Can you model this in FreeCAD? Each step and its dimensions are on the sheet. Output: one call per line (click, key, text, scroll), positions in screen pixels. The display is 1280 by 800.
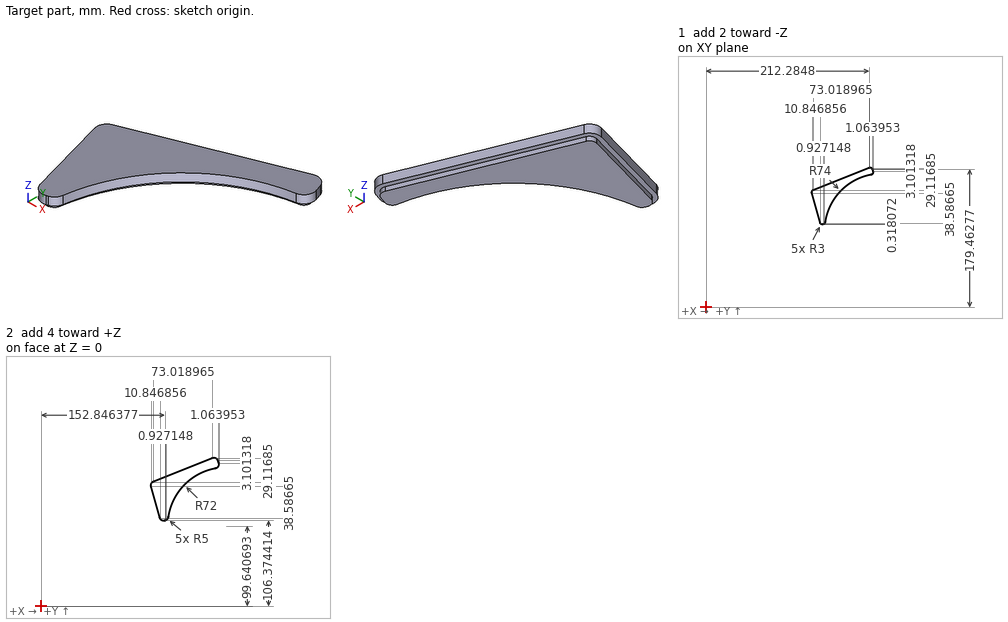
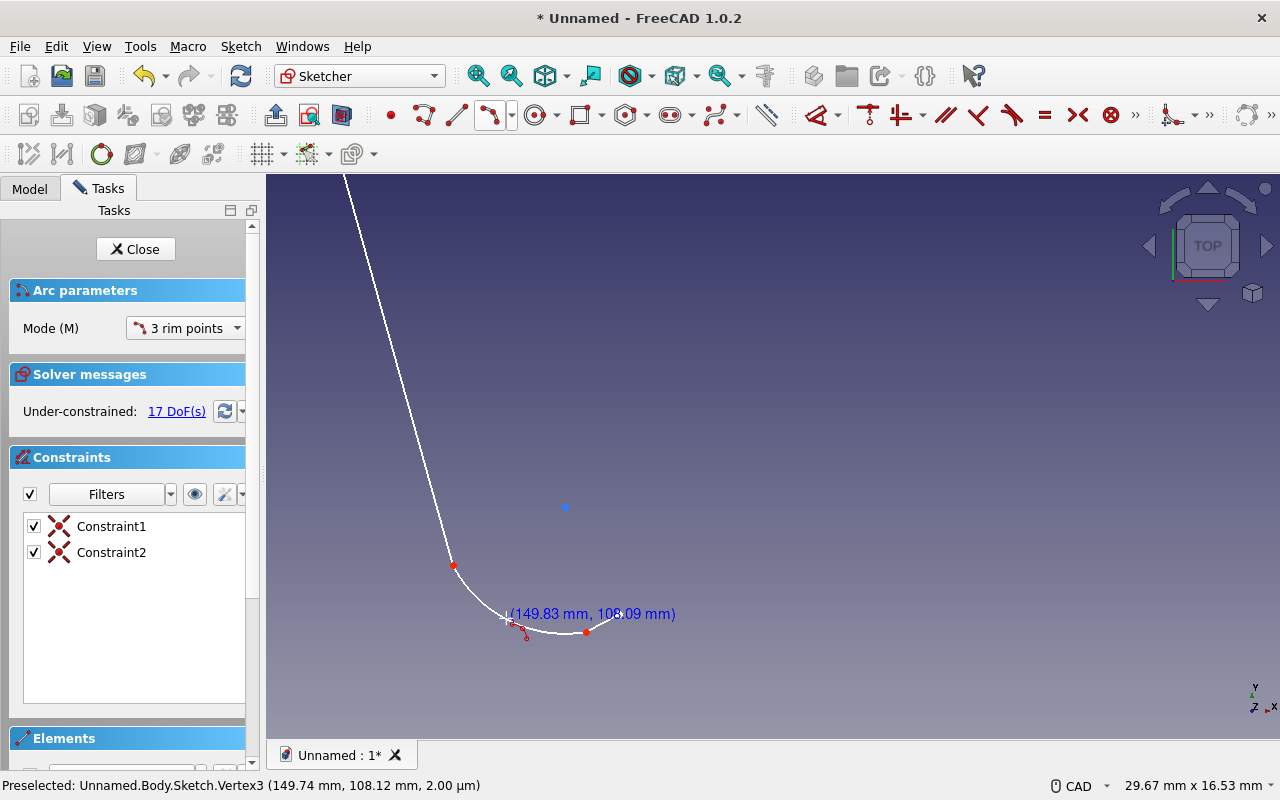
click(619, 614)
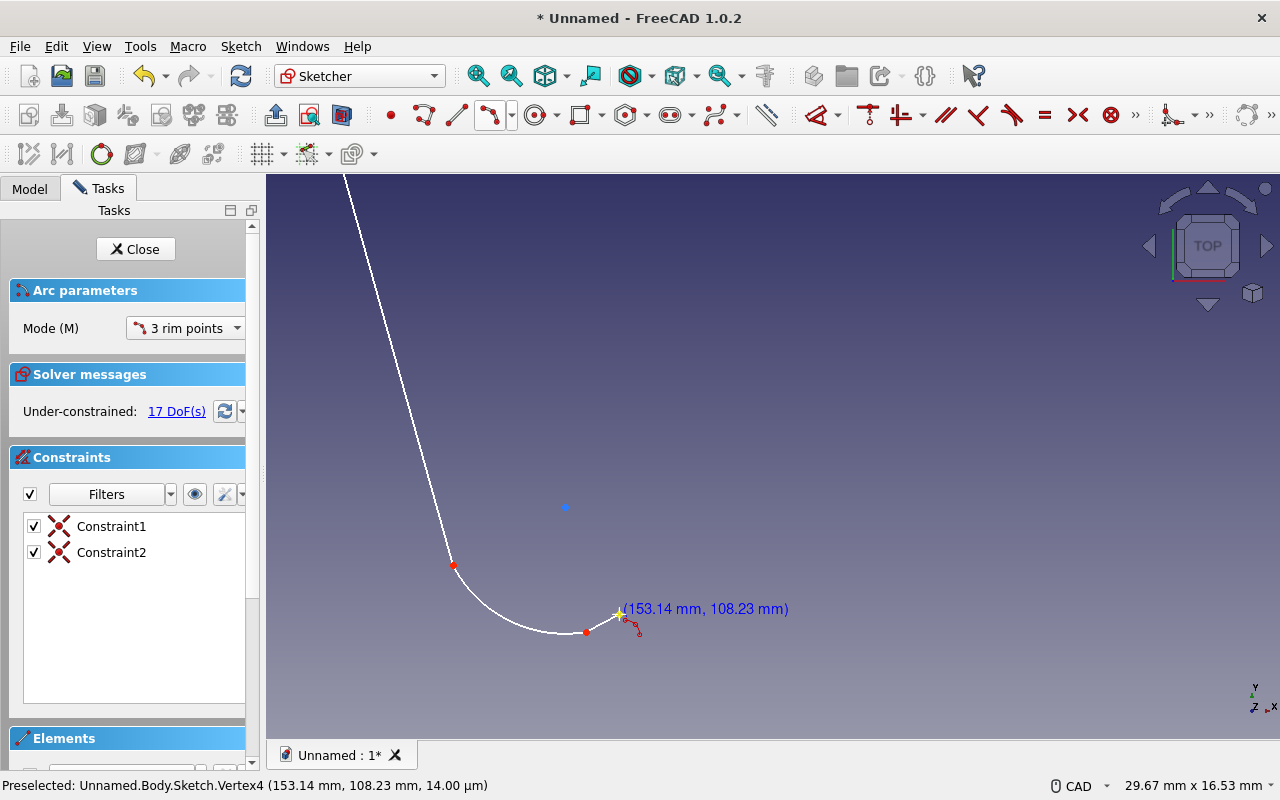
scroll(588, 626, down, 10)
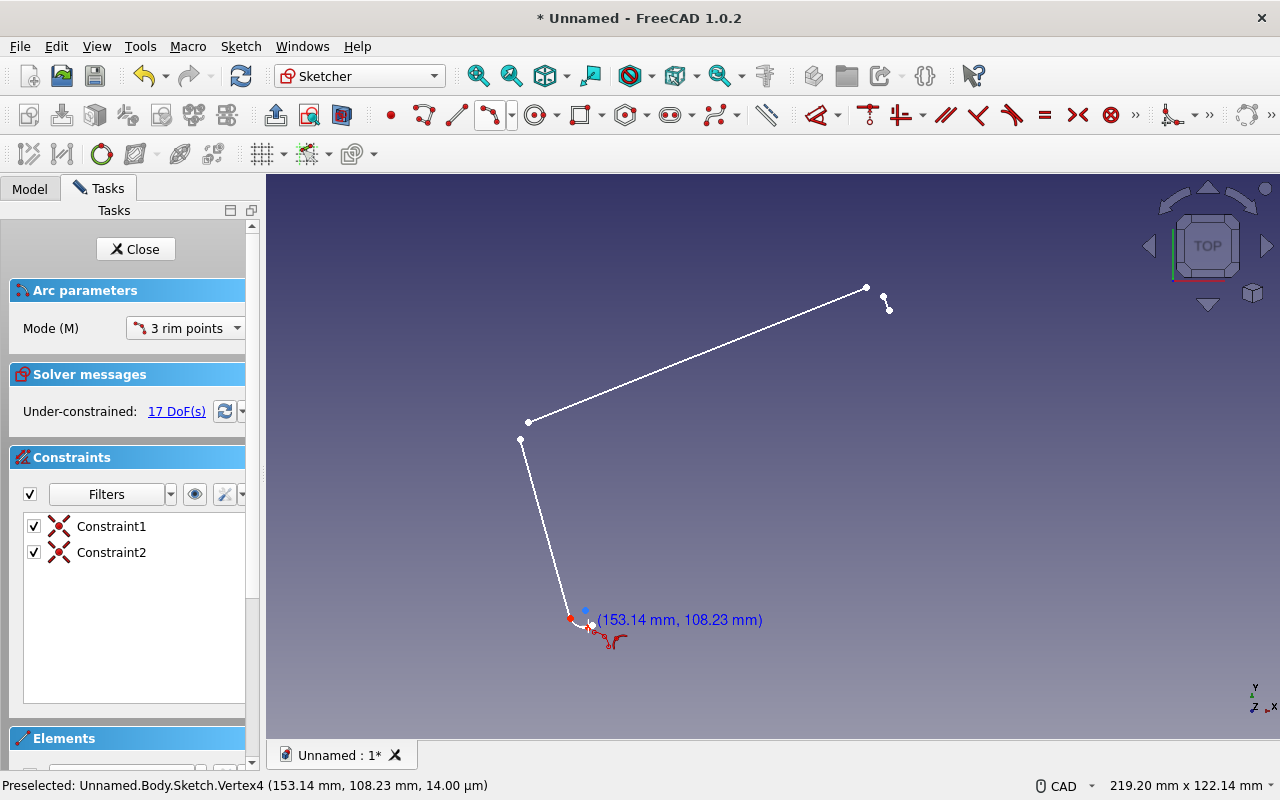
click(602, 614)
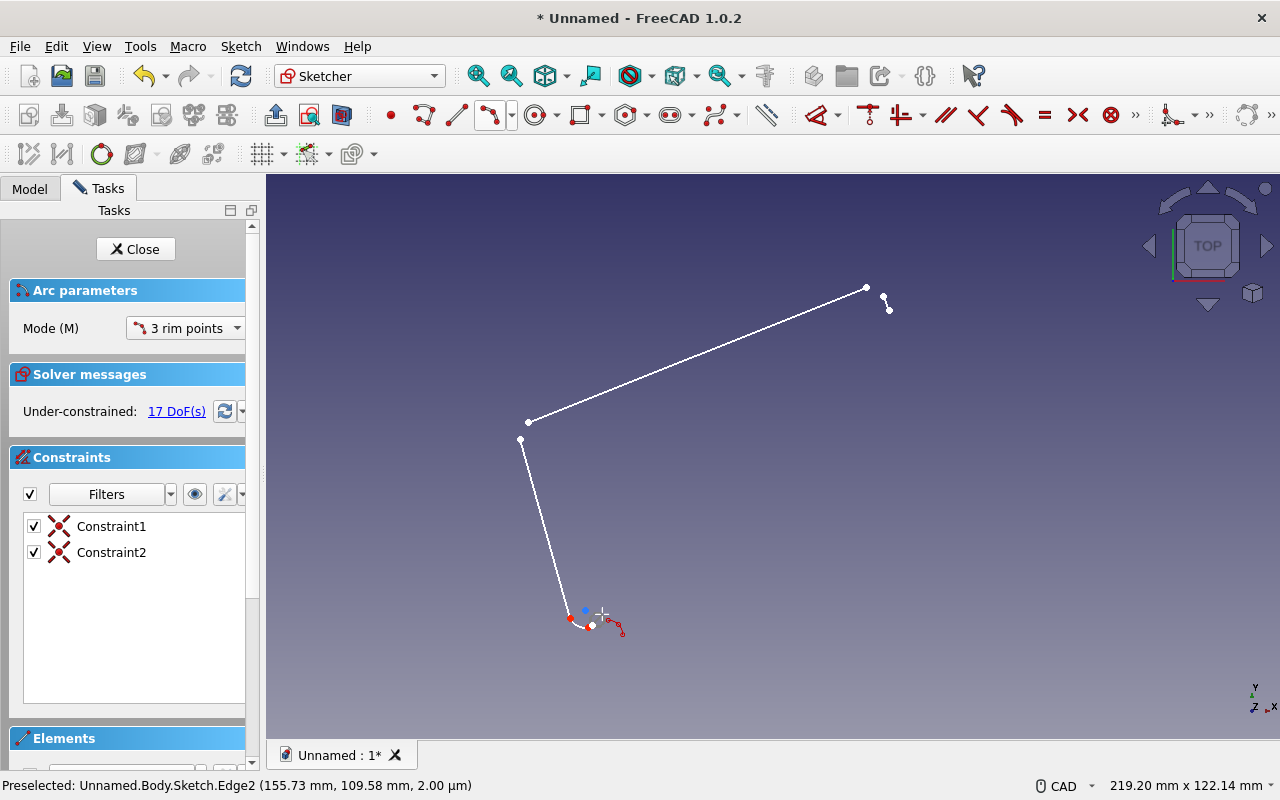
scroll(599, 621, up, 11)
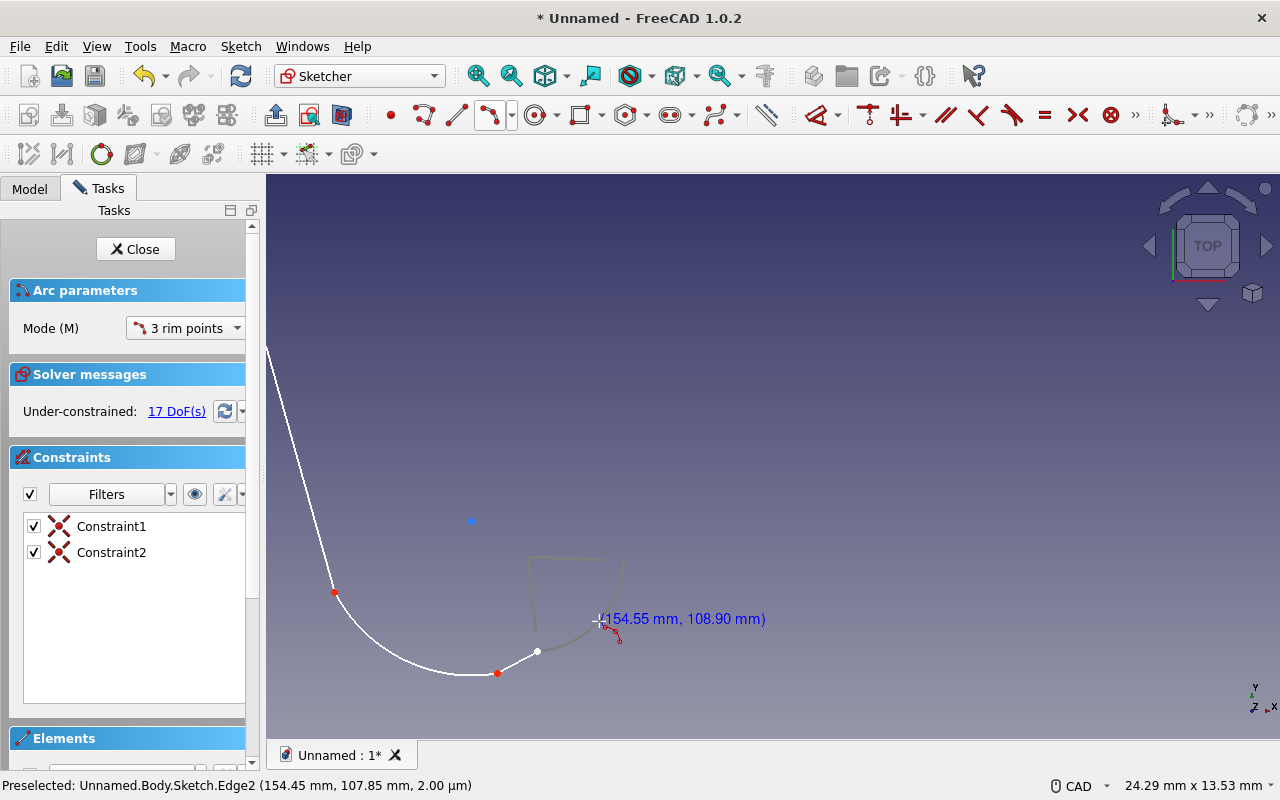
click(592, 612)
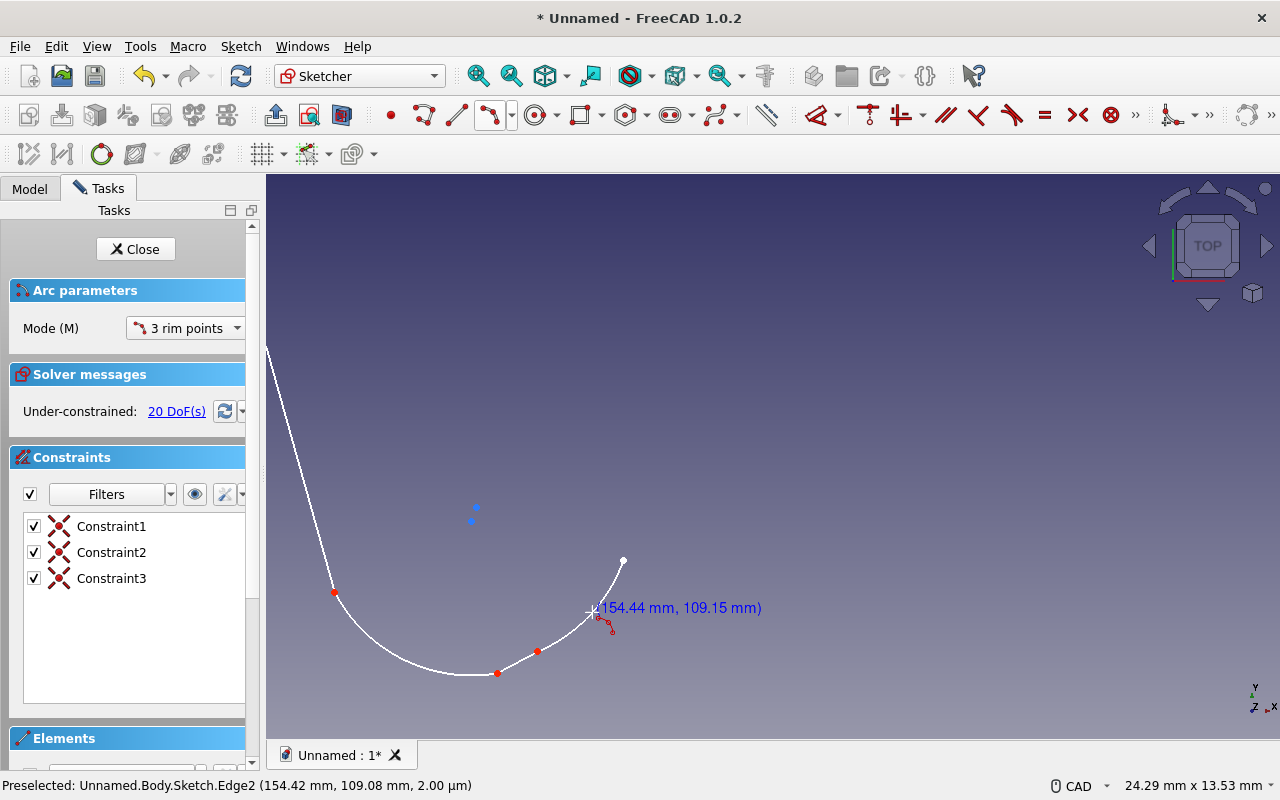
scroll(599, 621, down, 11)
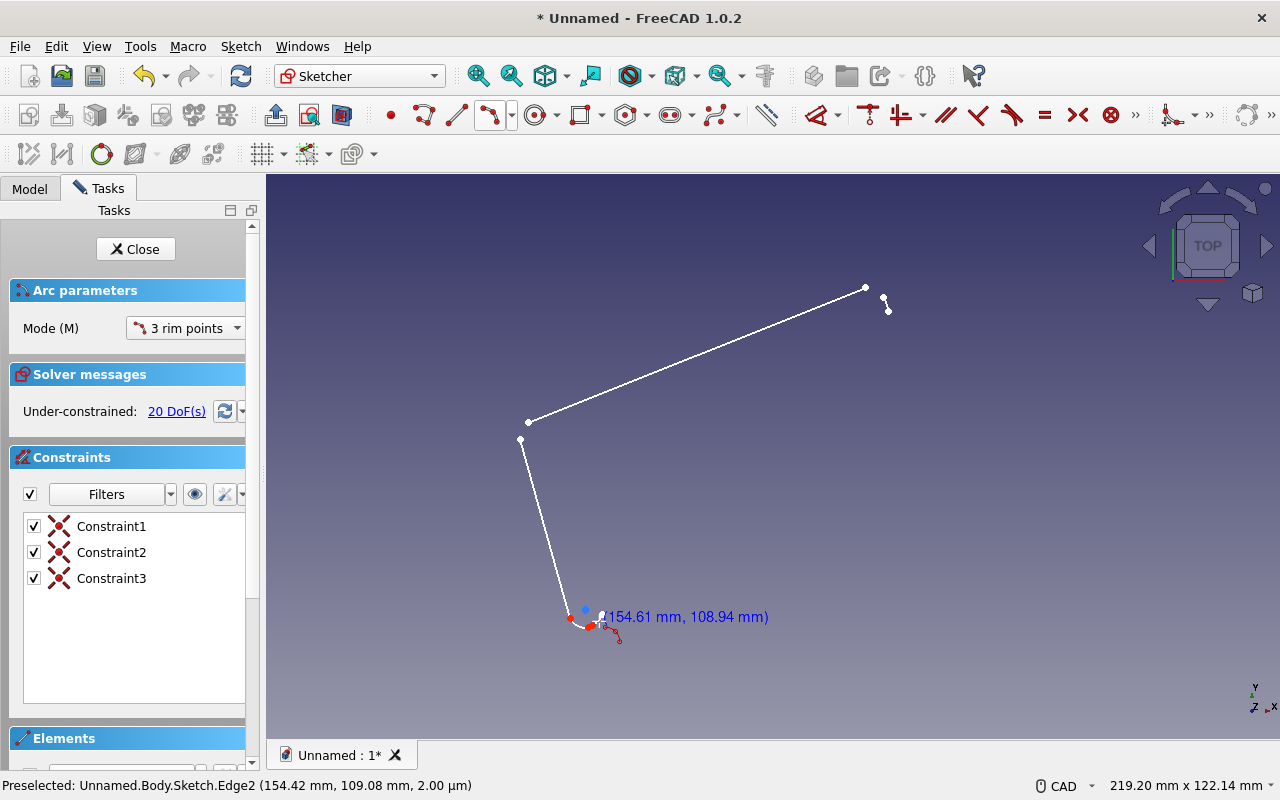
click(602, 615)
click(879, 328)
click(694, 427)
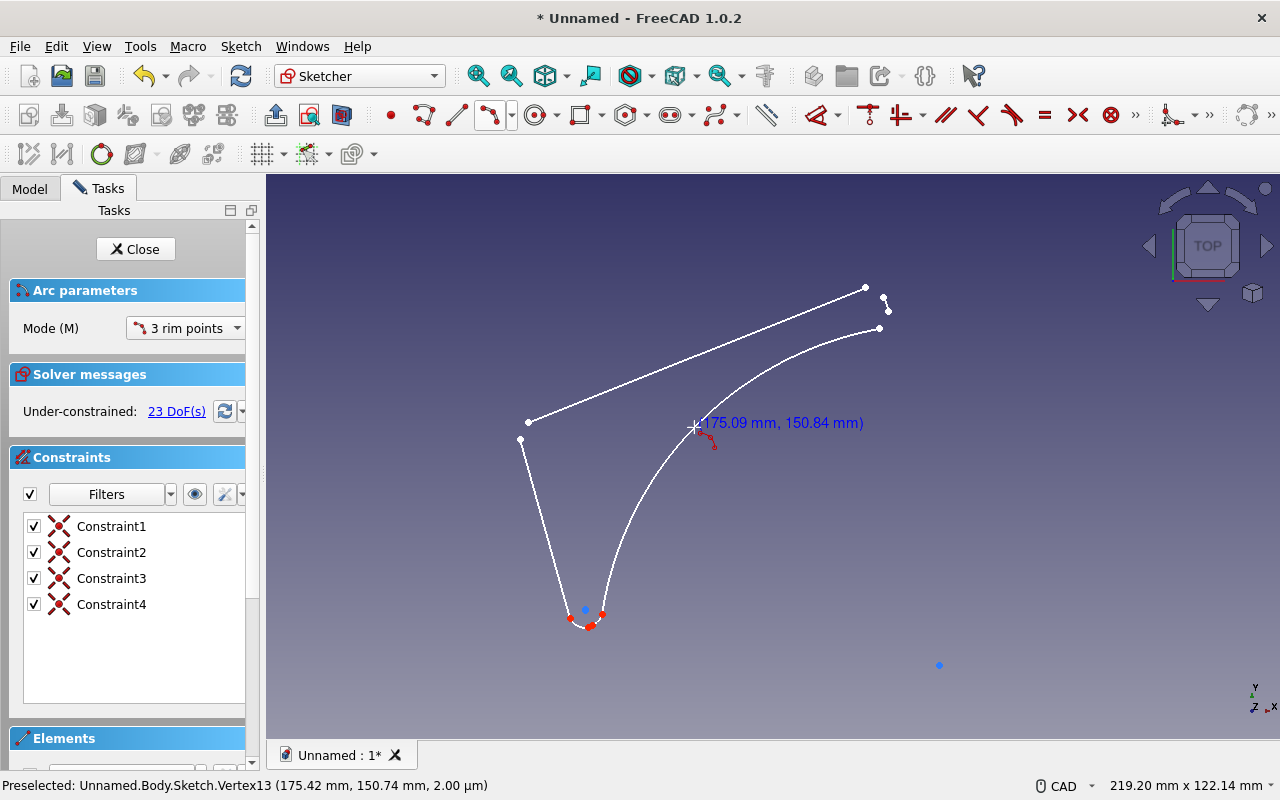
click(879, 329)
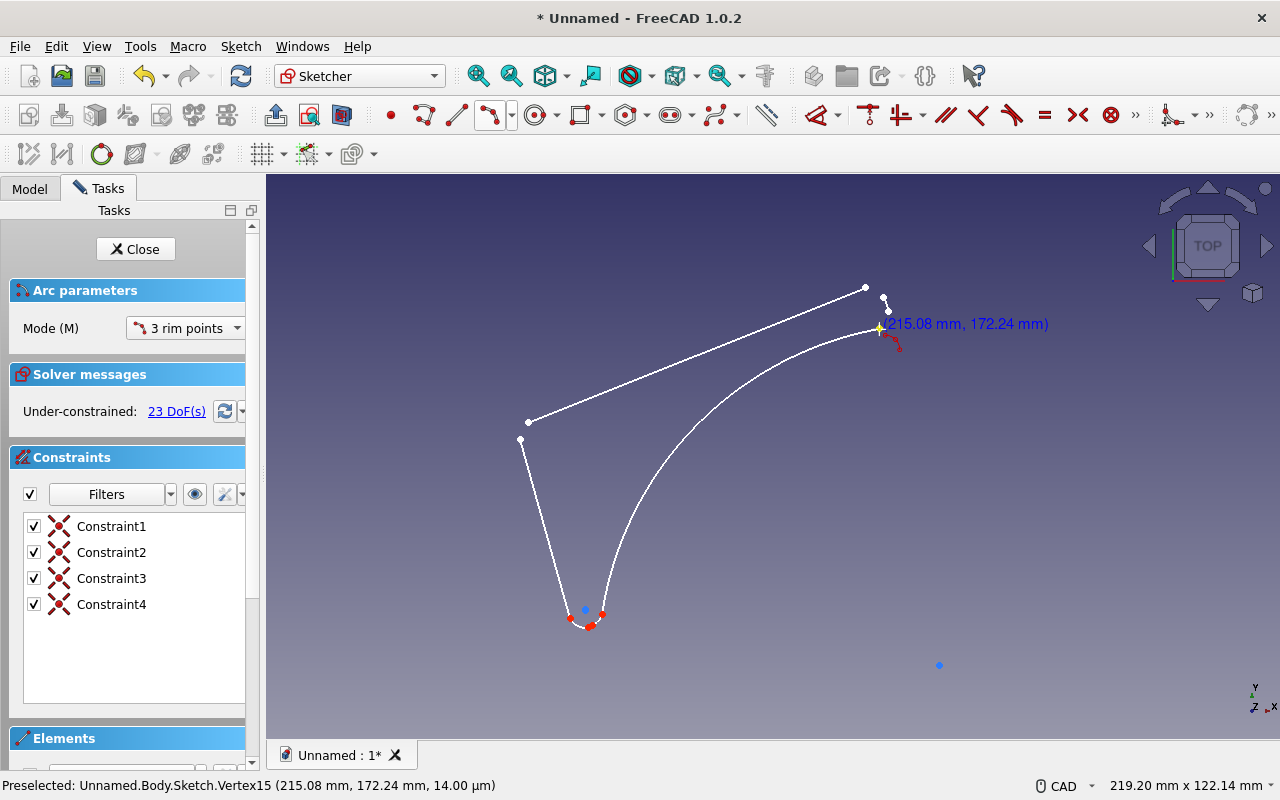
scroll(889, 310, up, 4)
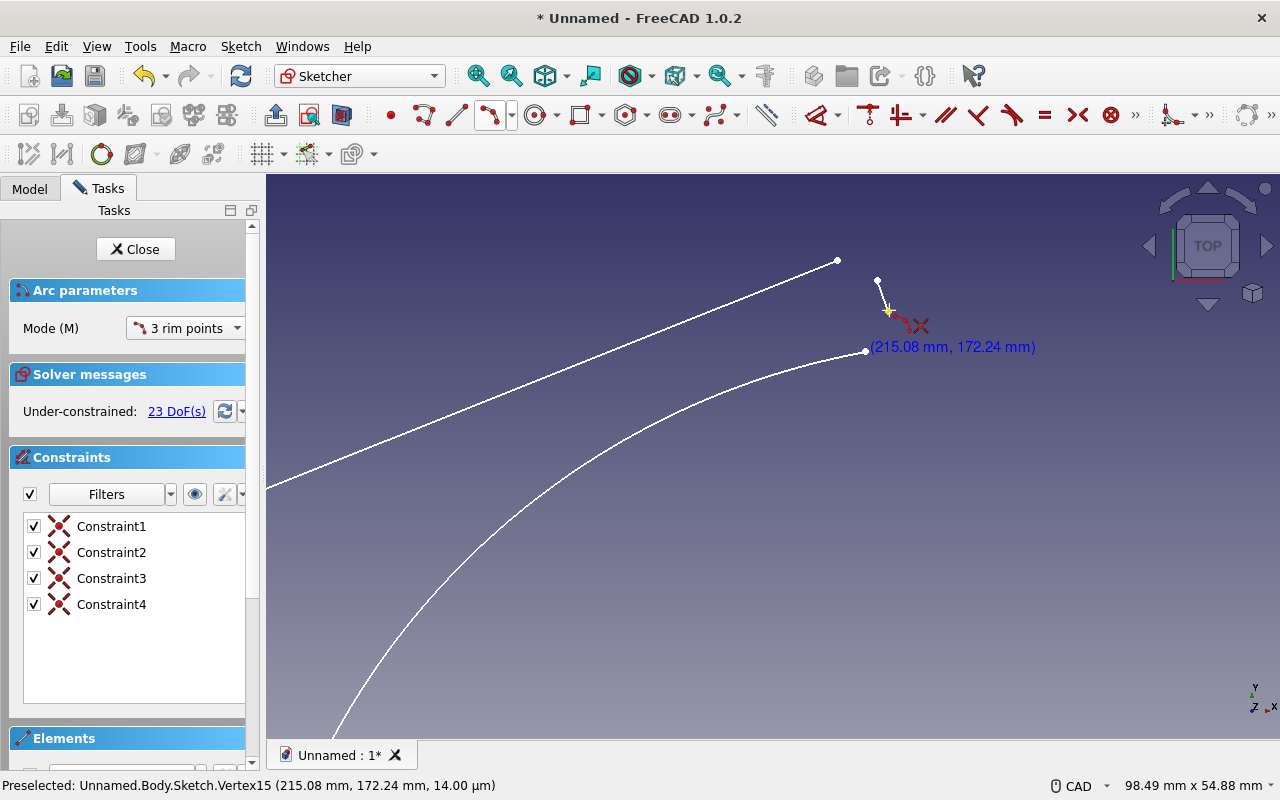
click(888, 312)